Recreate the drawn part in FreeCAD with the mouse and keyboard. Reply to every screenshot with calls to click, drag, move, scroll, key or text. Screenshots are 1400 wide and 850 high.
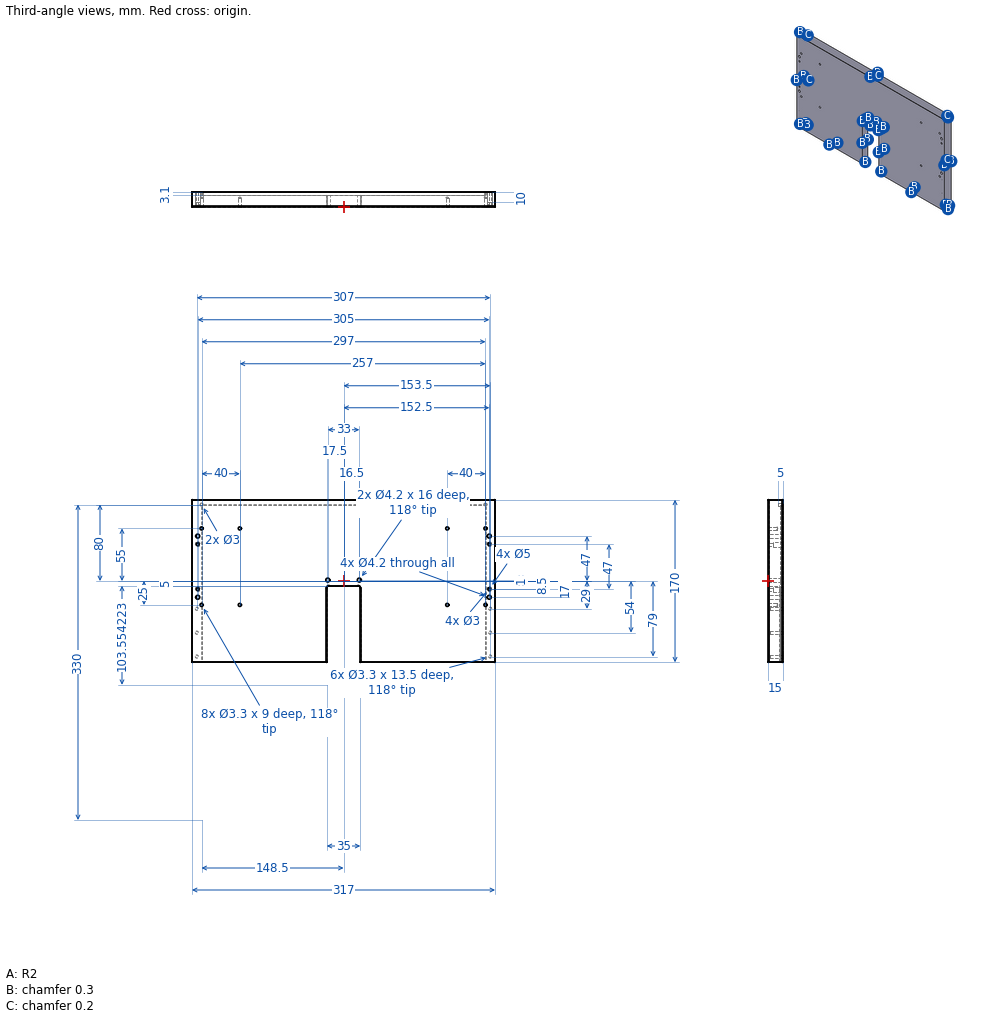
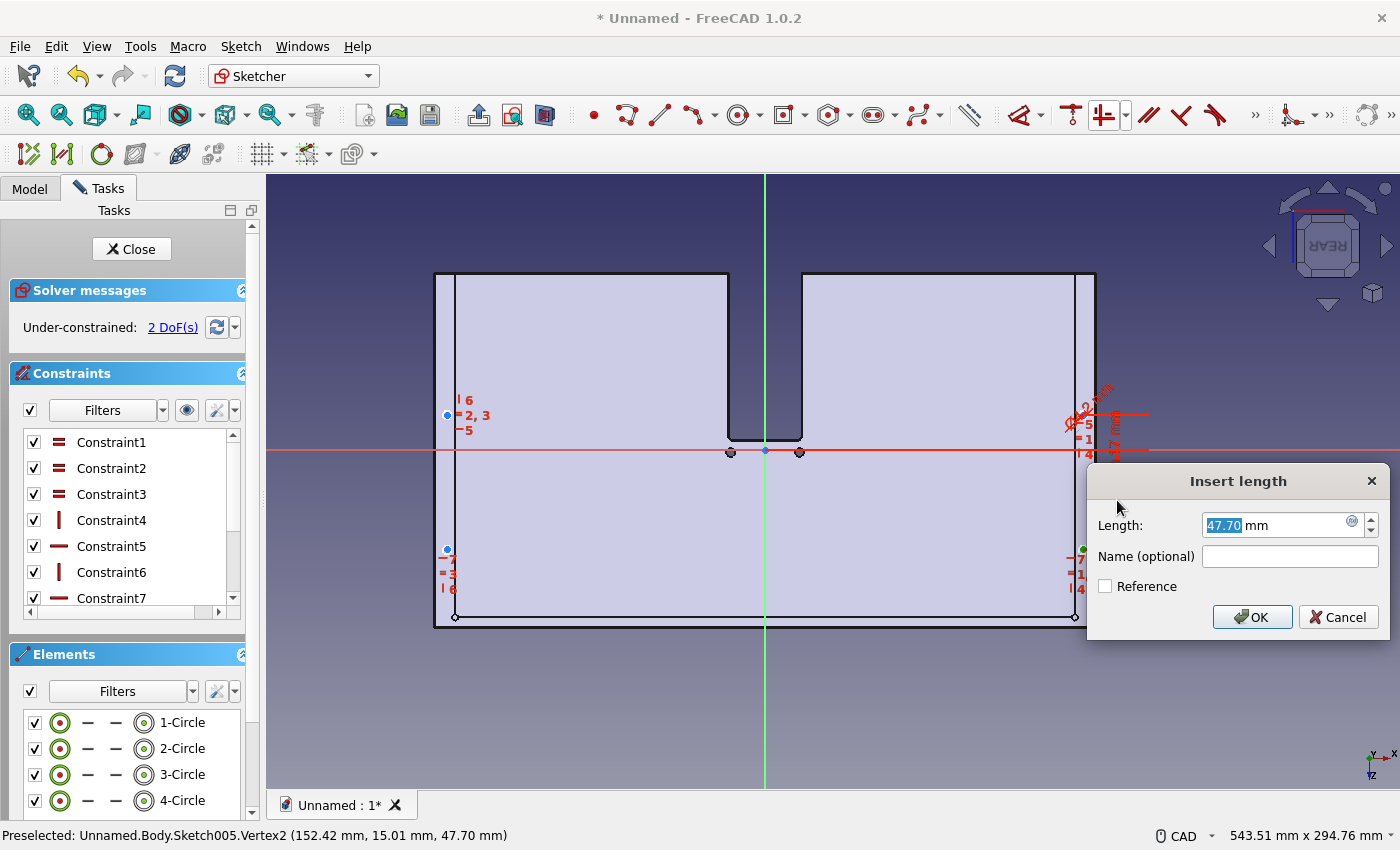
text(47)
key(Return)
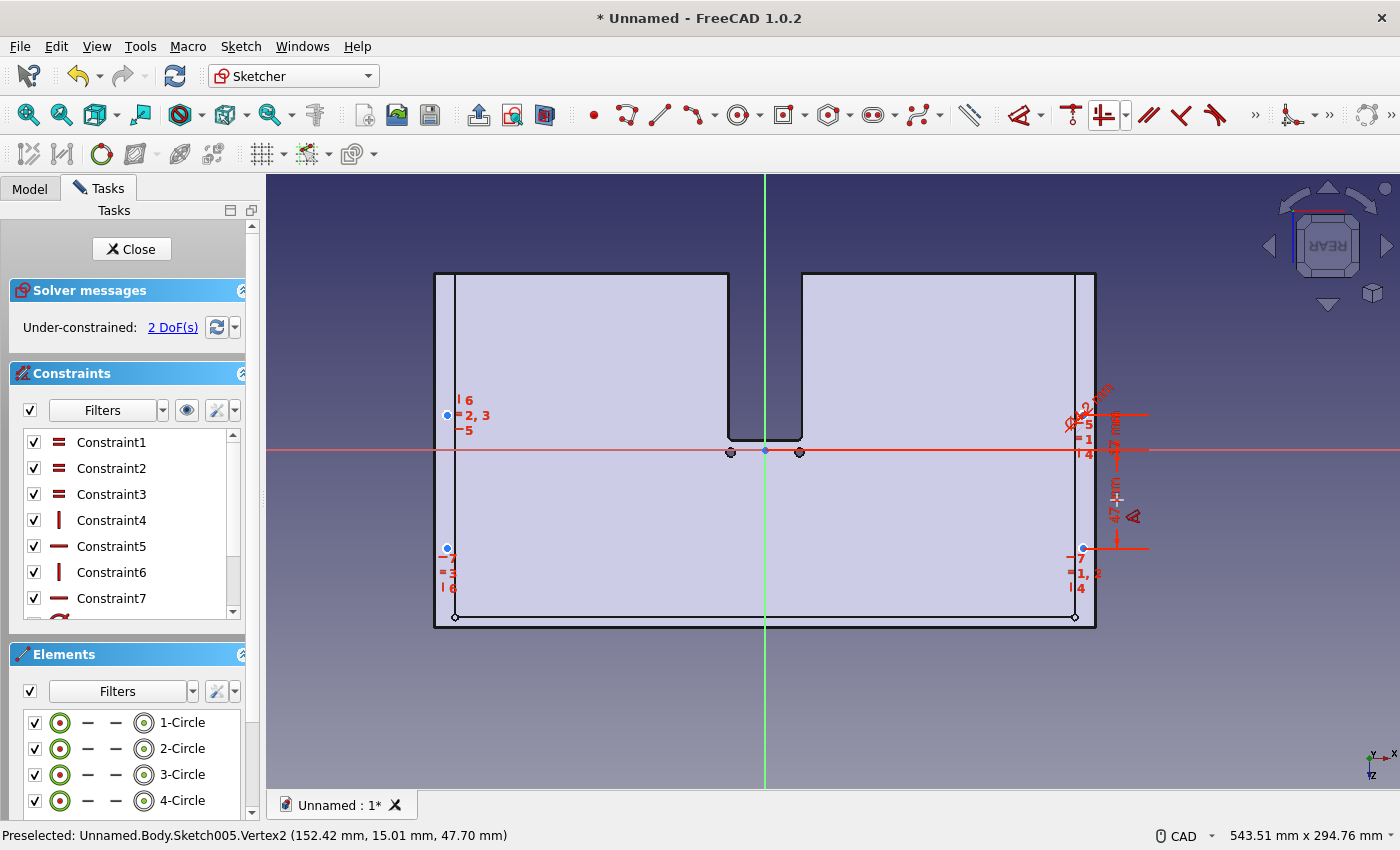
click(1083, 415)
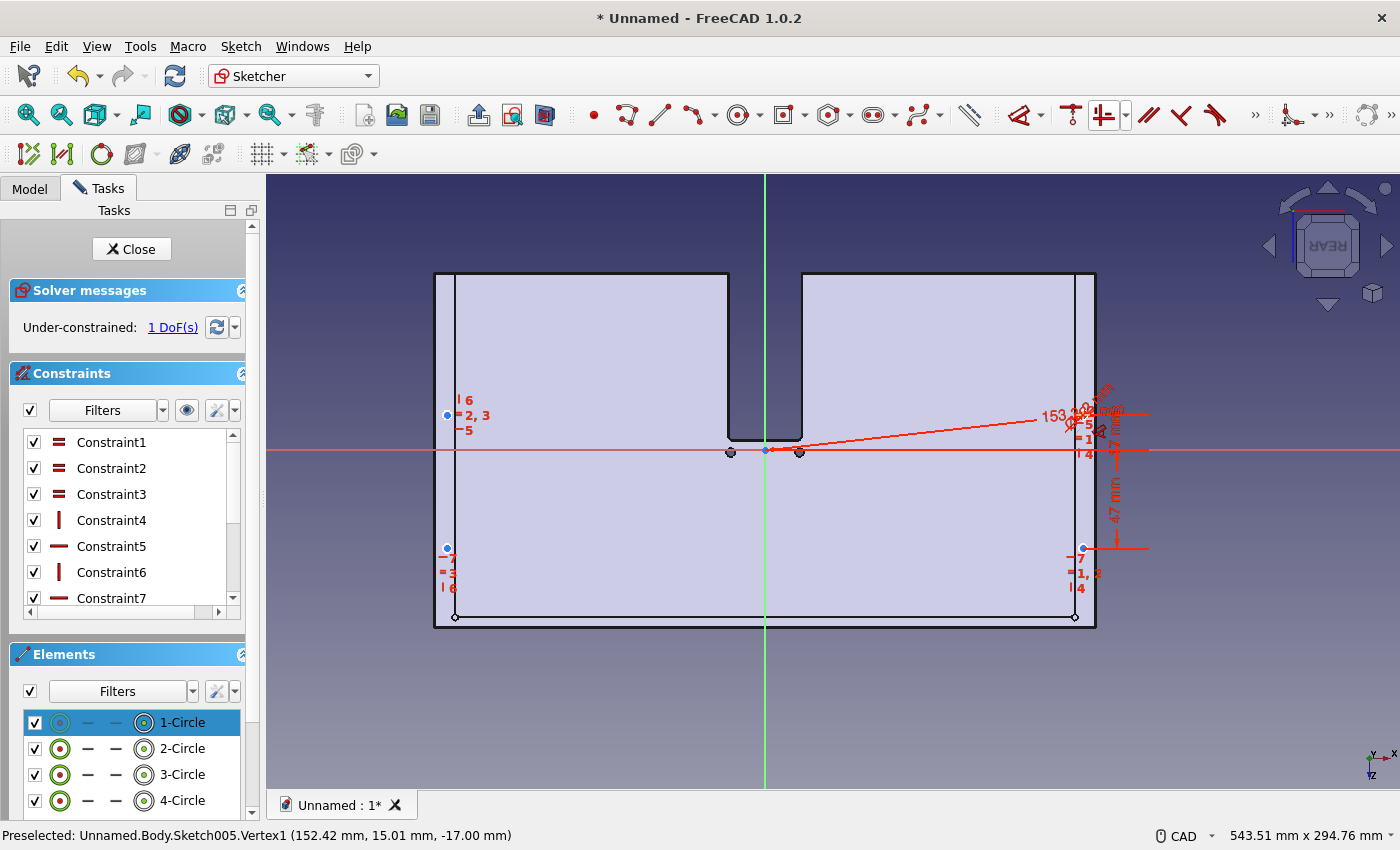
click(447, 415)
click(619, 381)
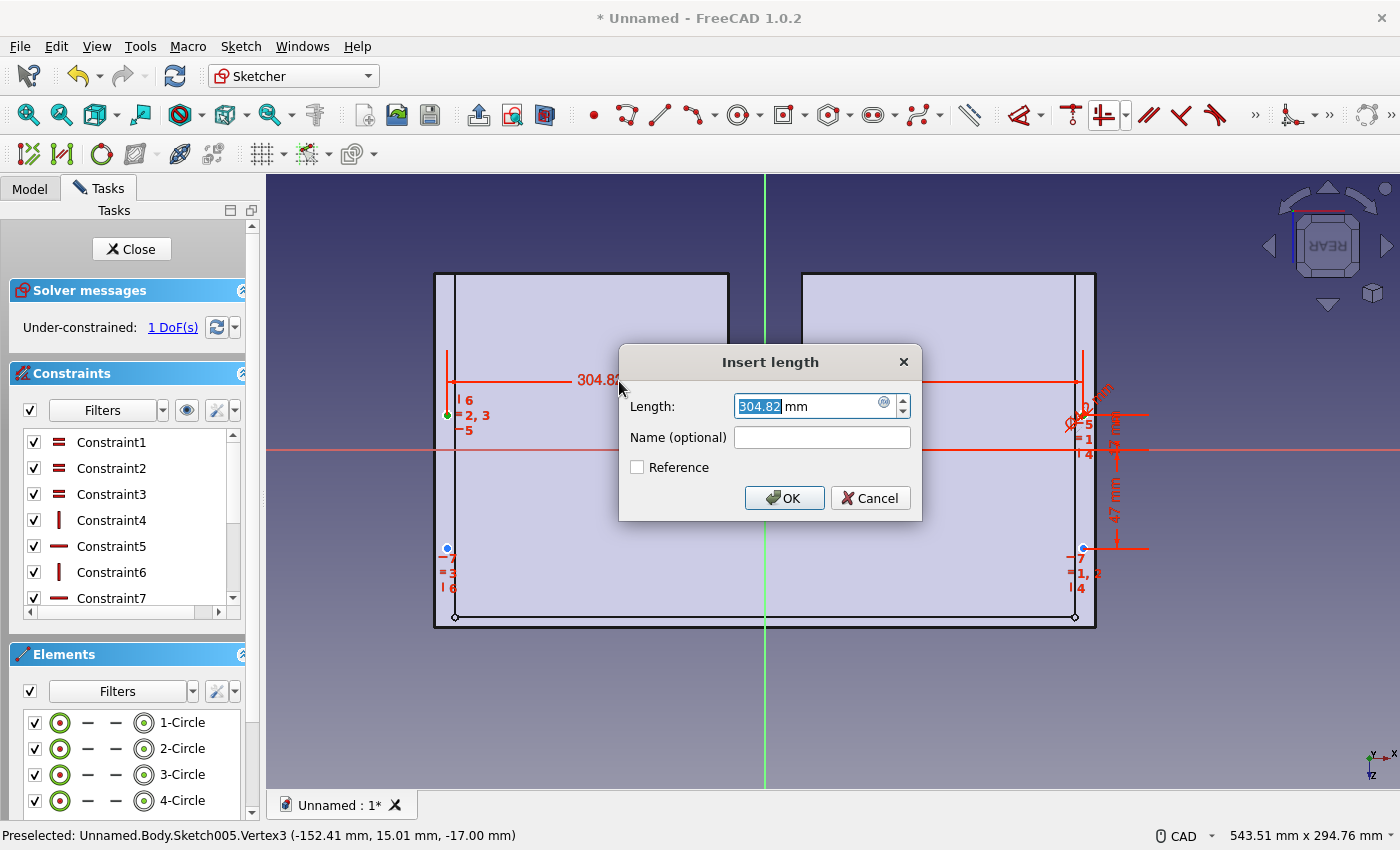
text(305)
key(Return)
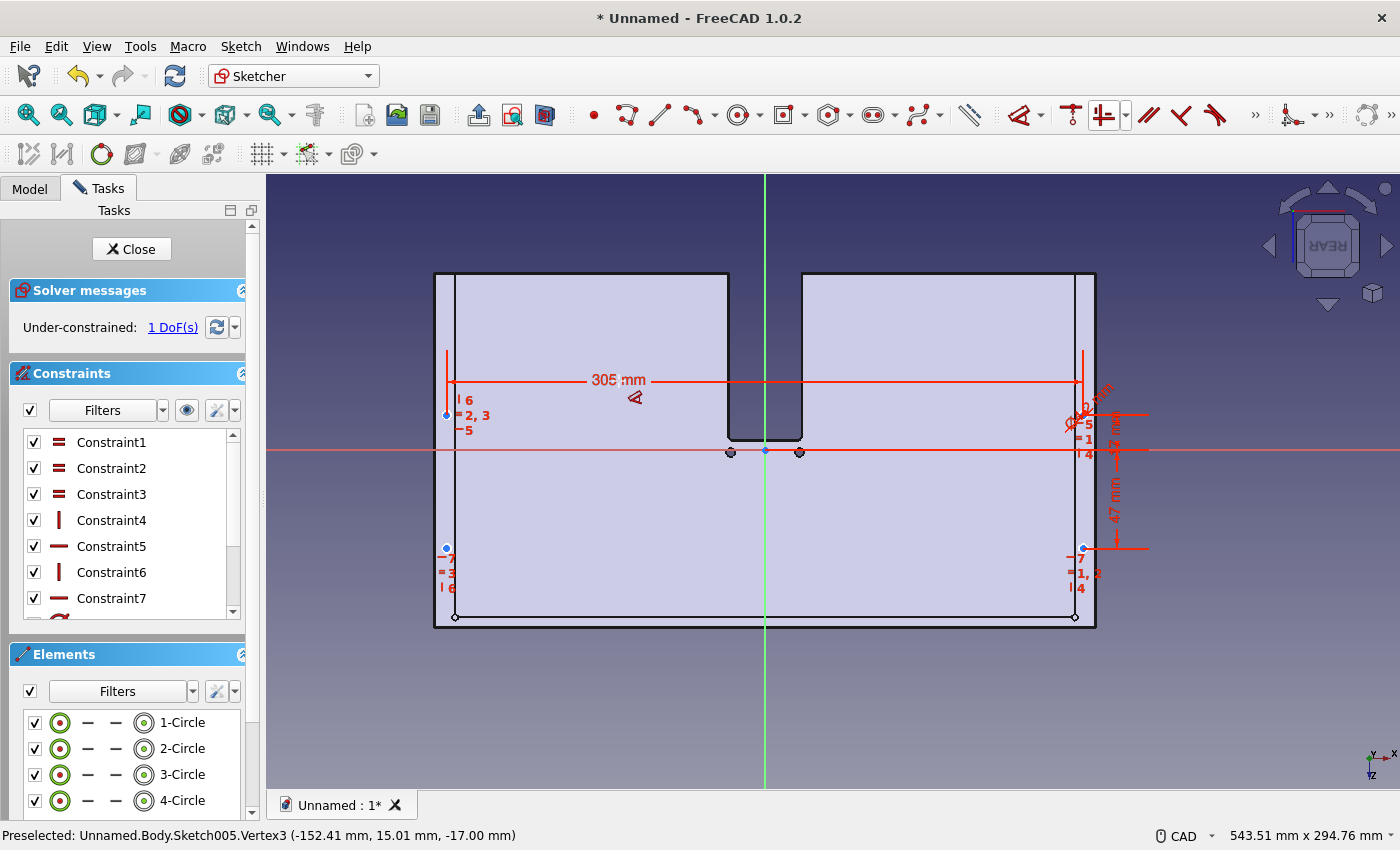
click(1083, 415)
click(924, 381)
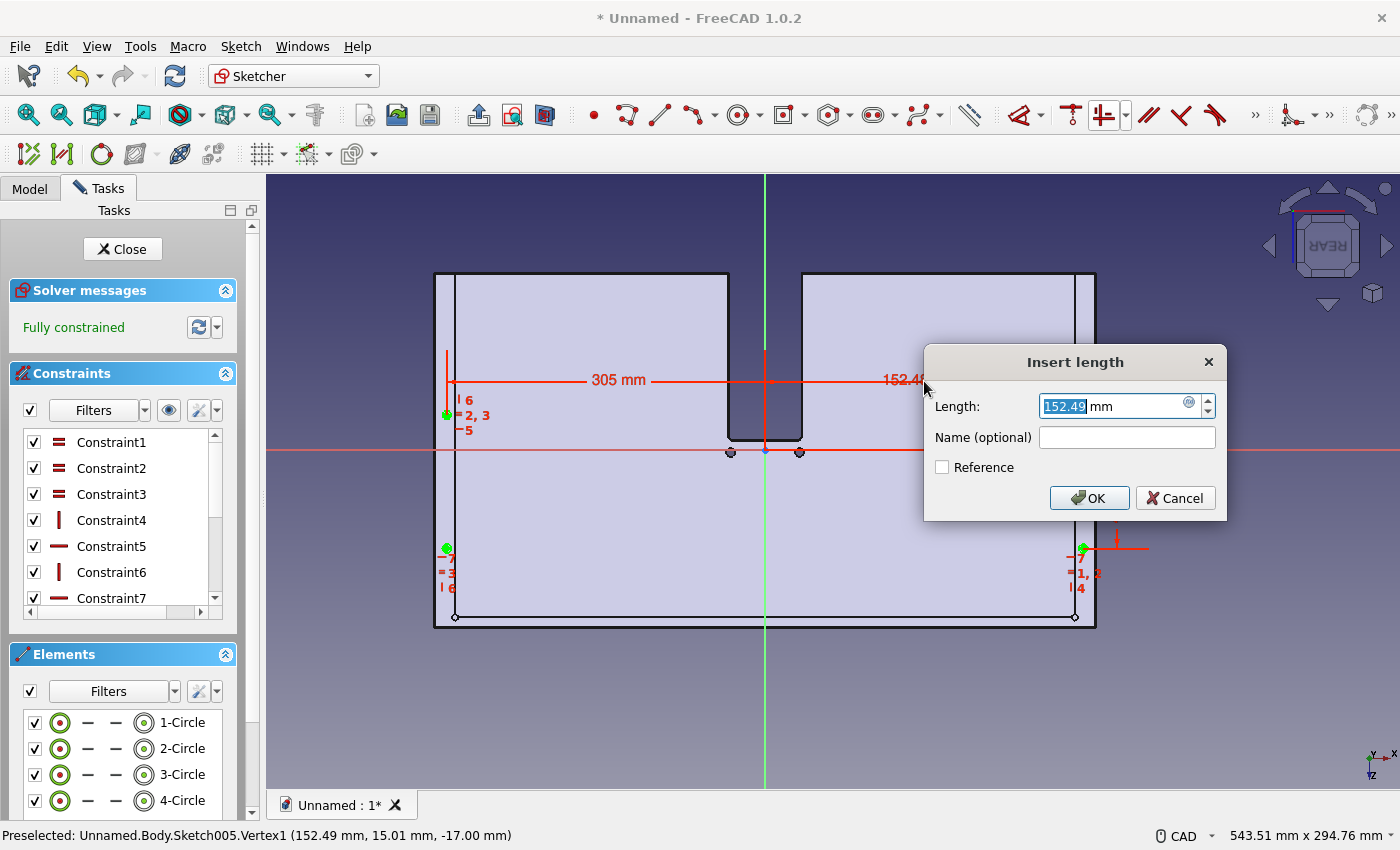
text(152.5)
key(Return)
key(Escape)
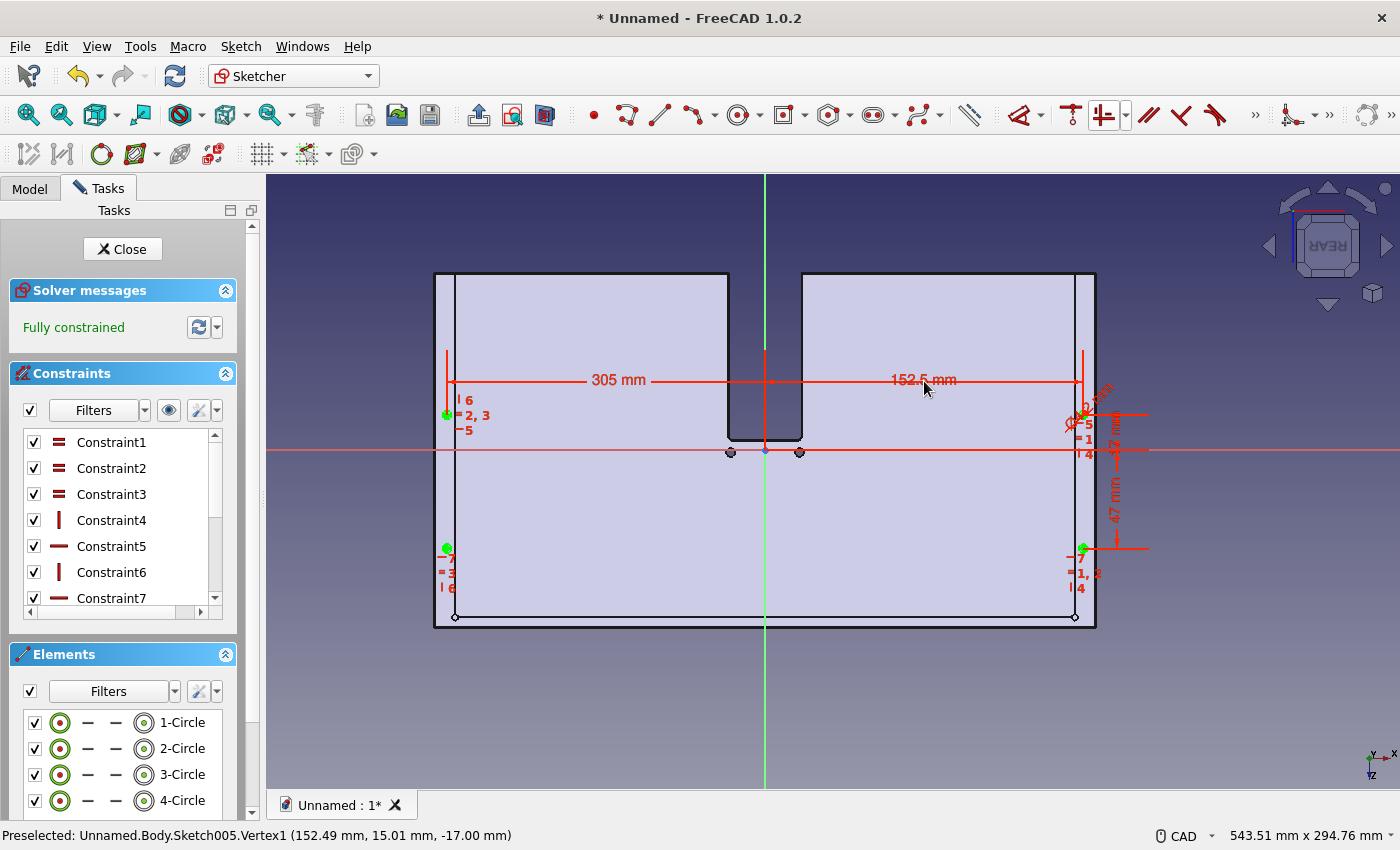
click(123, 249)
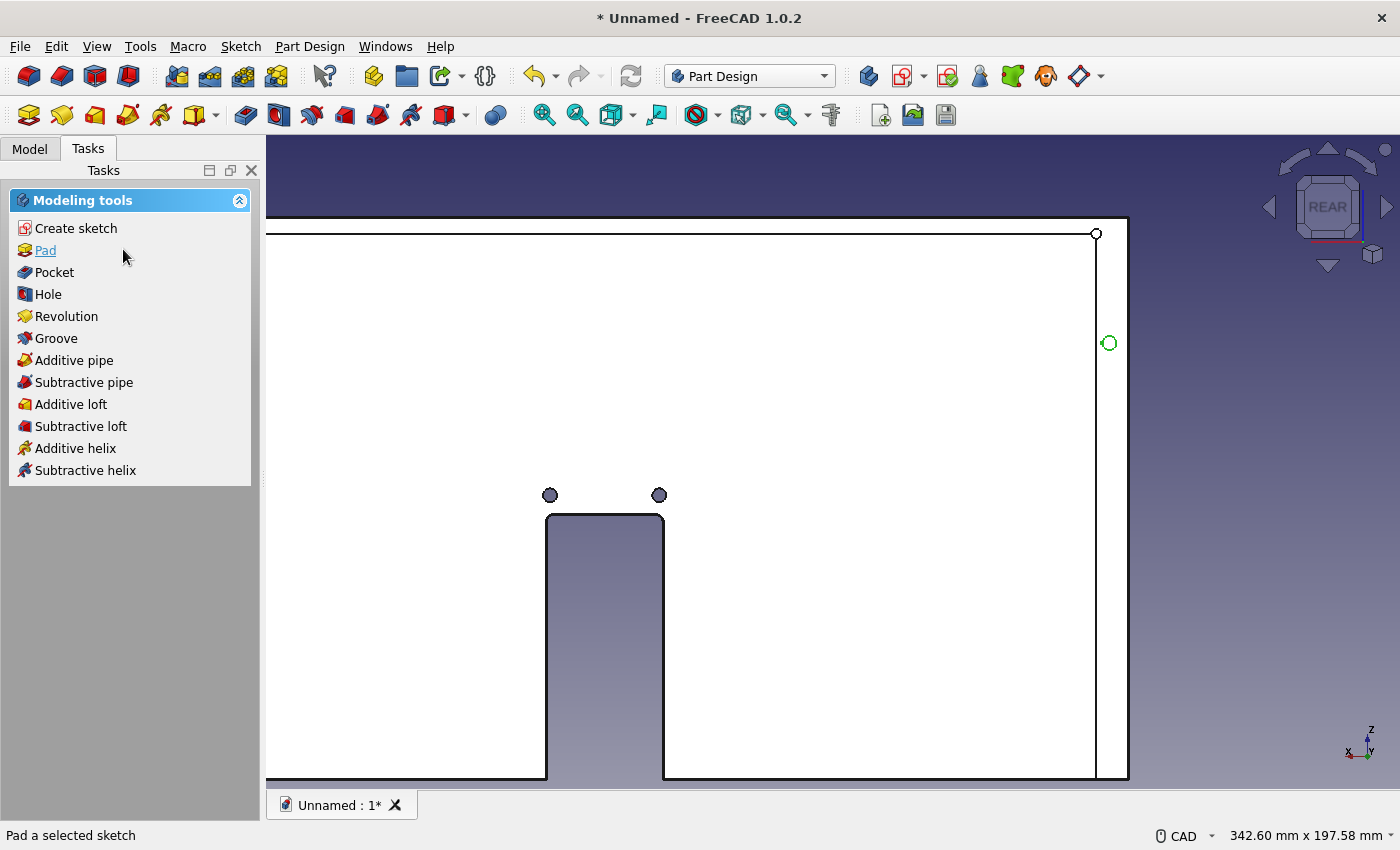
click(279, 116)